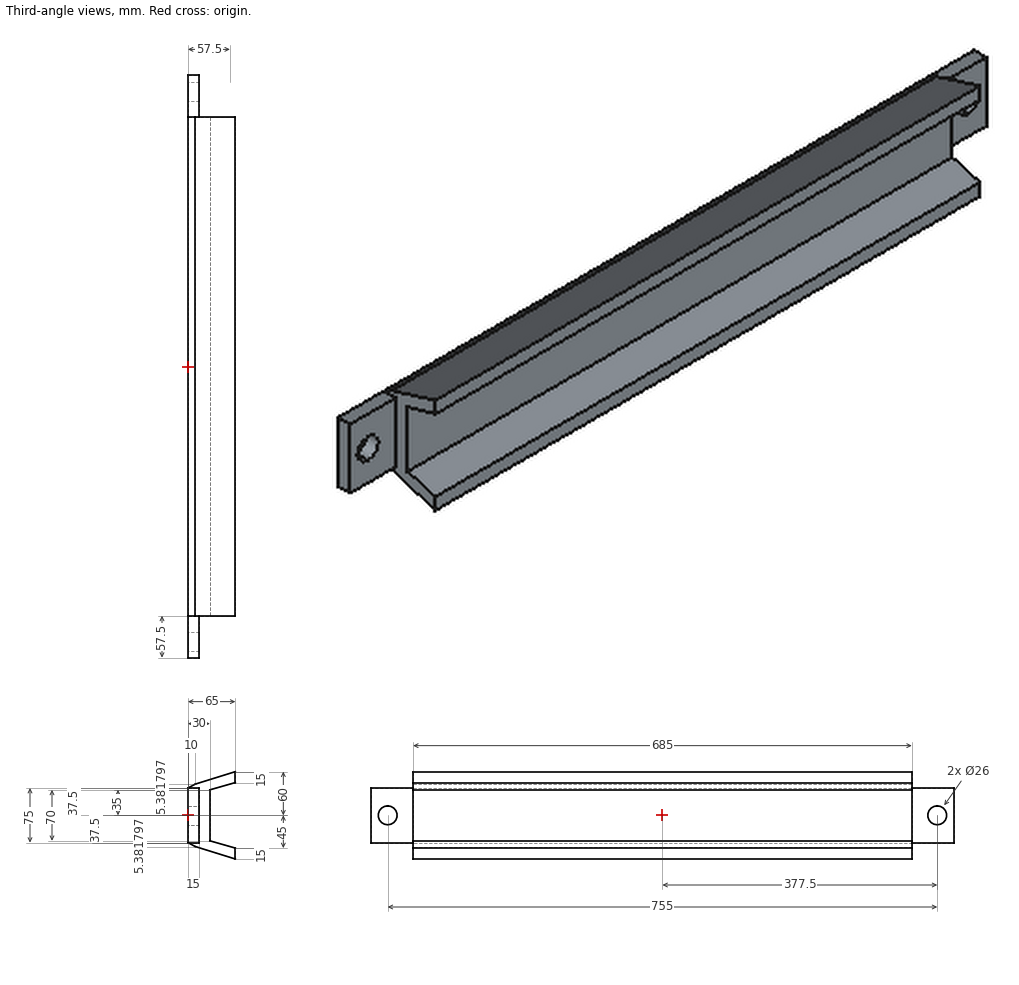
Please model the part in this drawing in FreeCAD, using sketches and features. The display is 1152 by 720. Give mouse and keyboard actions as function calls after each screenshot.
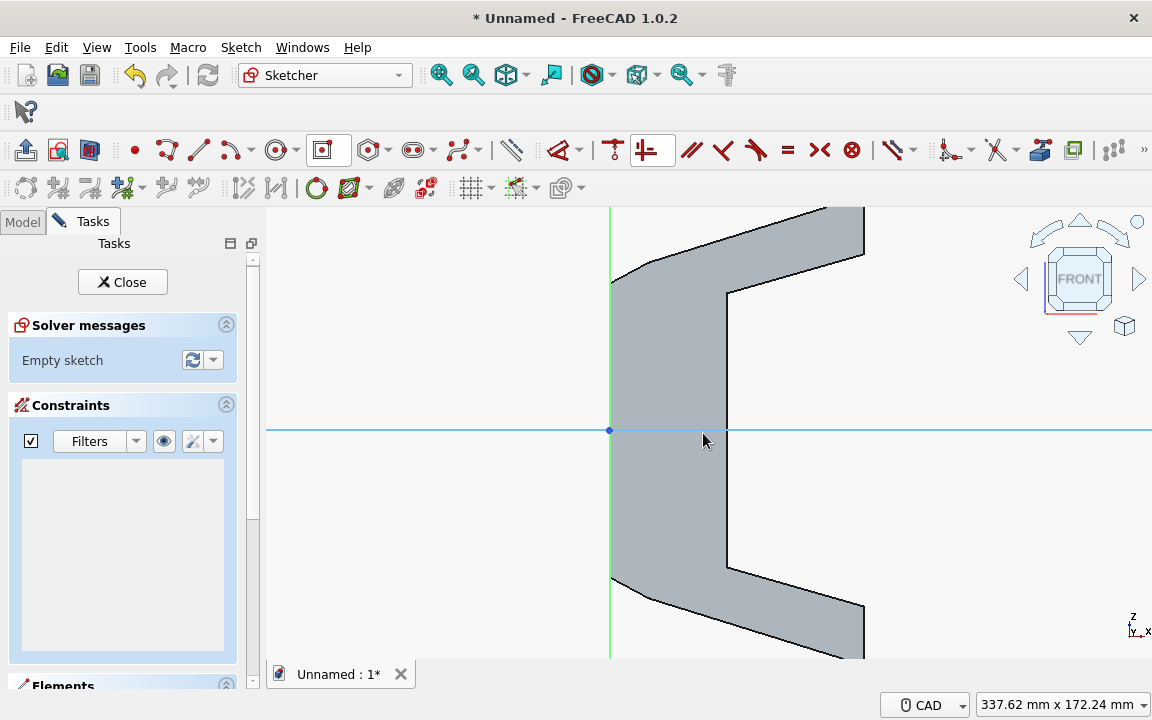
click(346, 150)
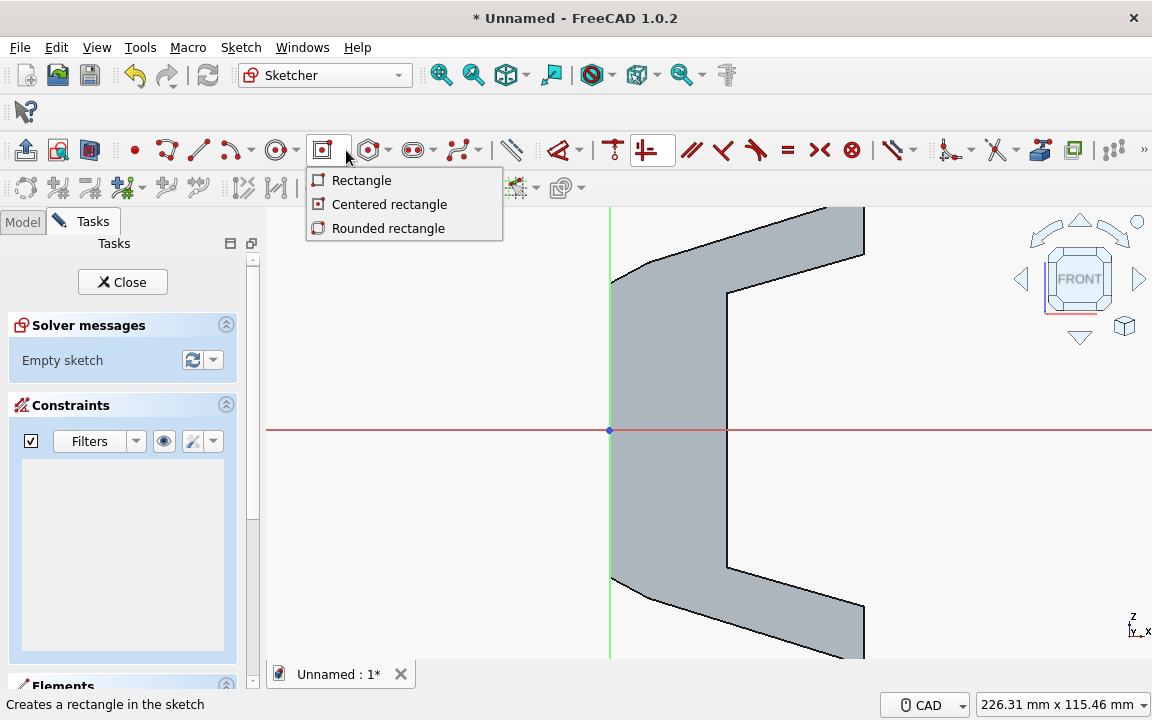
click(404, 180)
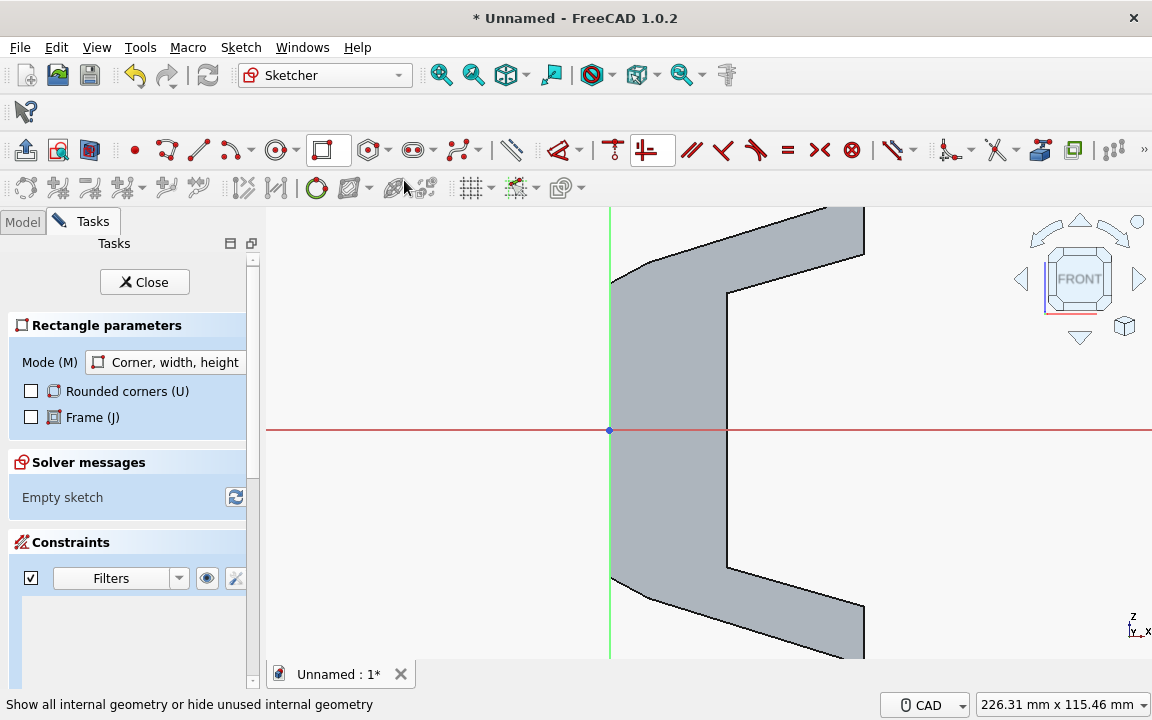
click(610, 284)
click(668, 577)
key(Escape)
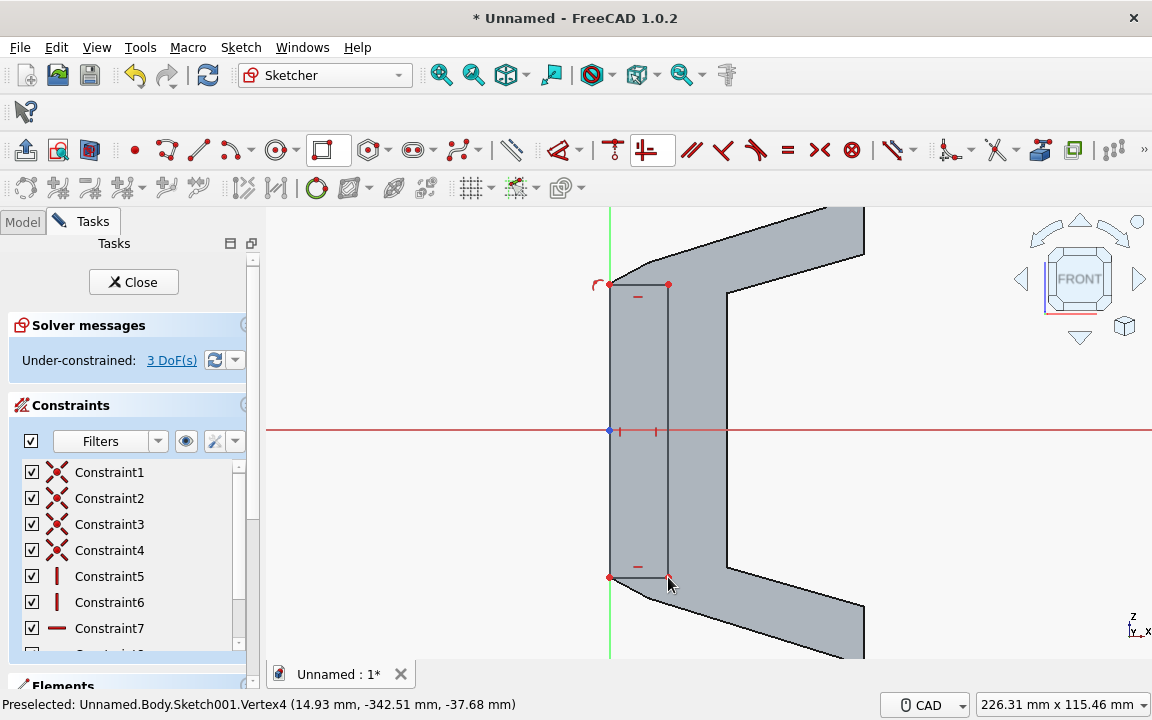
click(558, 150)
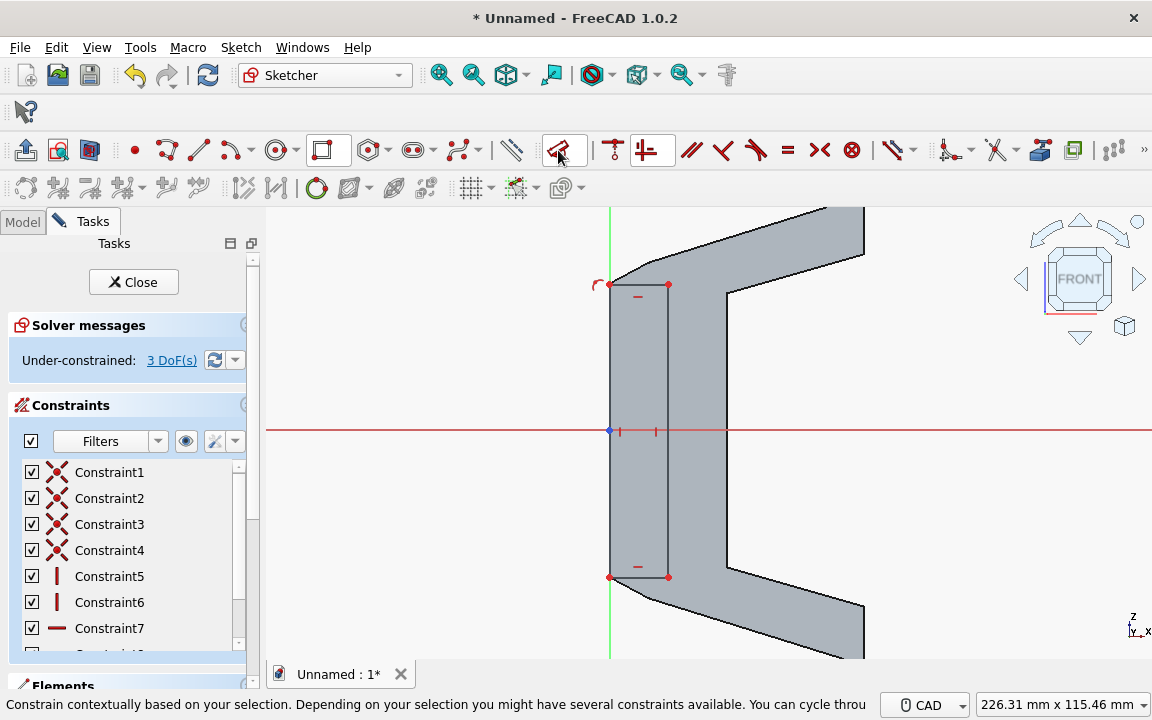
click(610, 373)
click(576, 364)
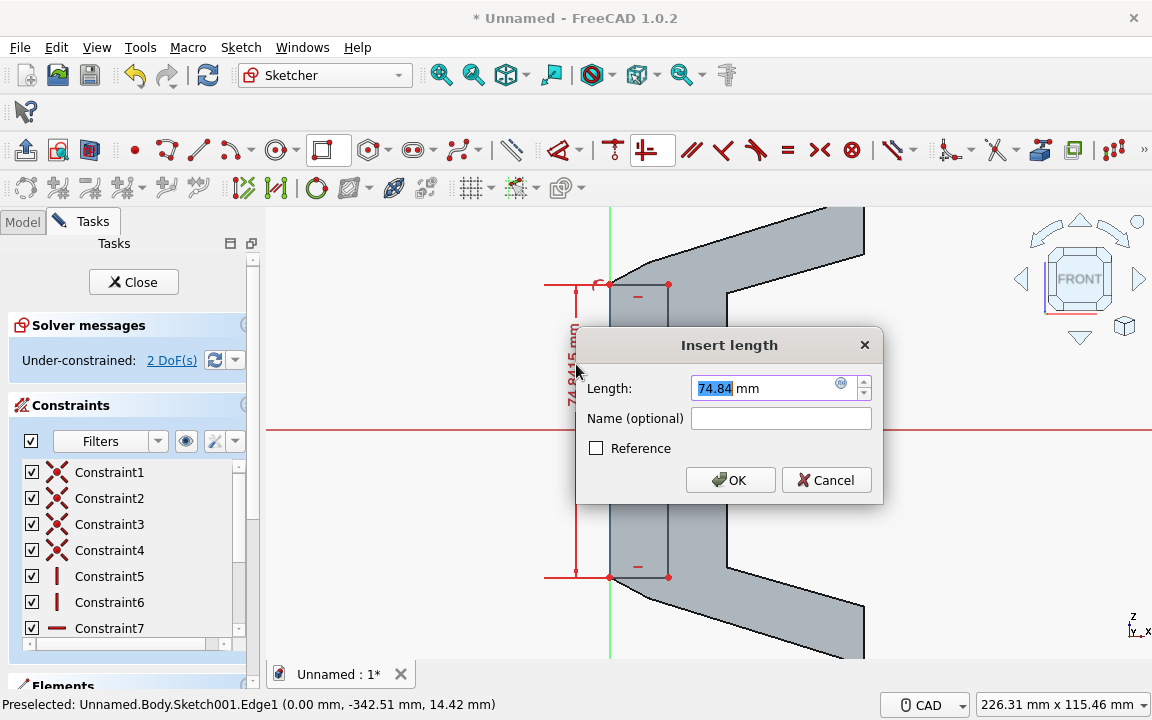
text(75)
key(Return)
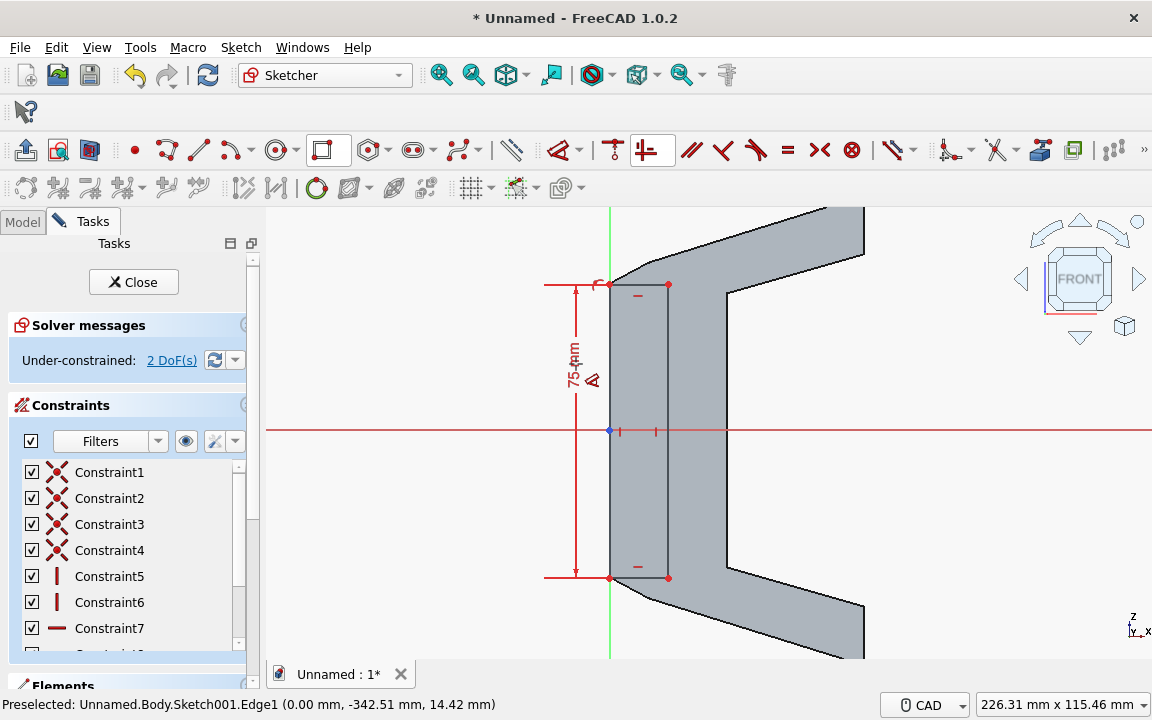
click(627, 578)
click(639, 612)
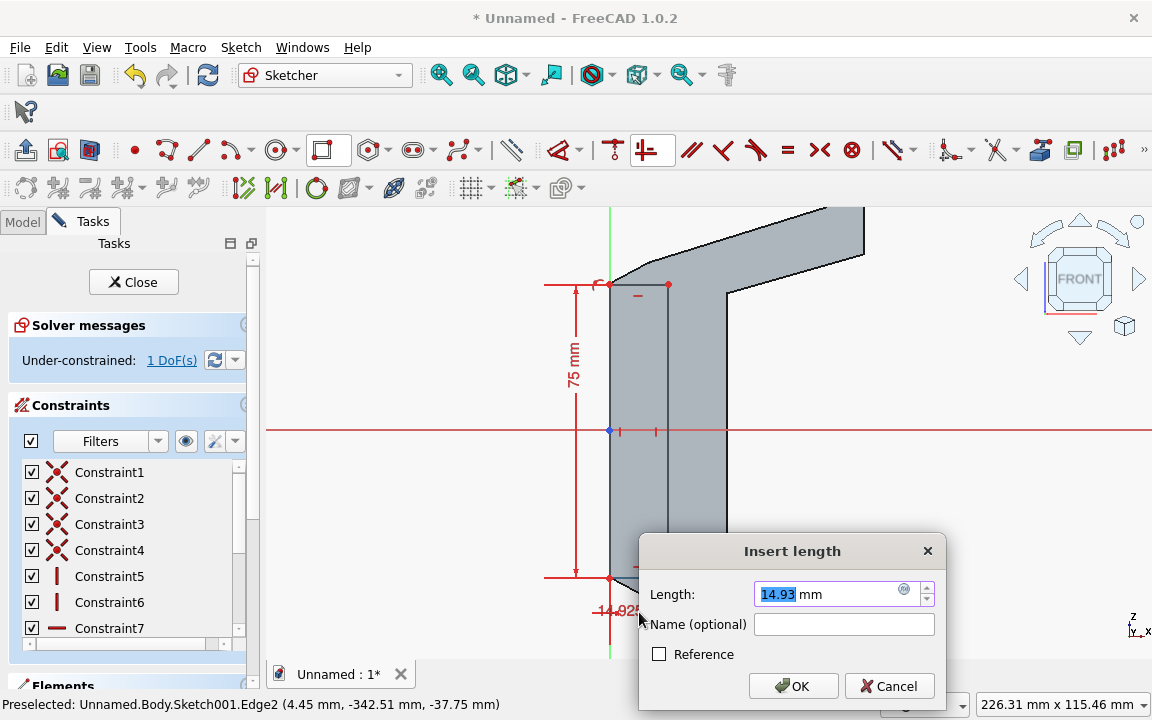
text(15)
key(Return)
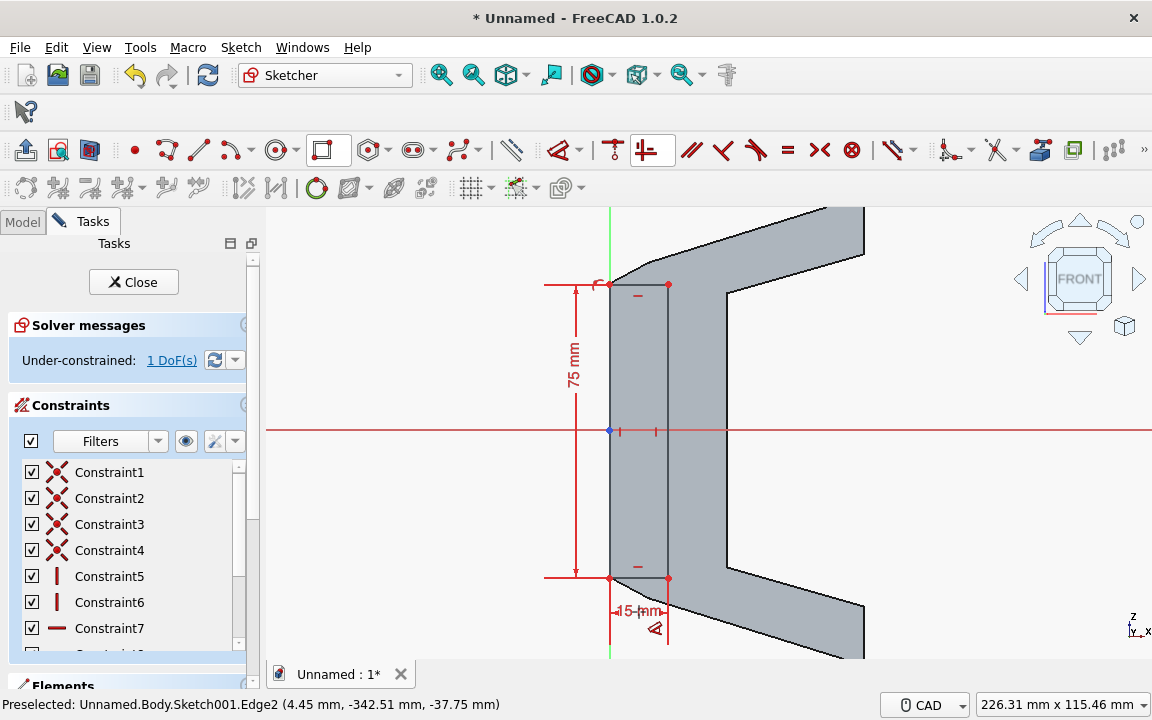
click(610, 285)
click(576, 324)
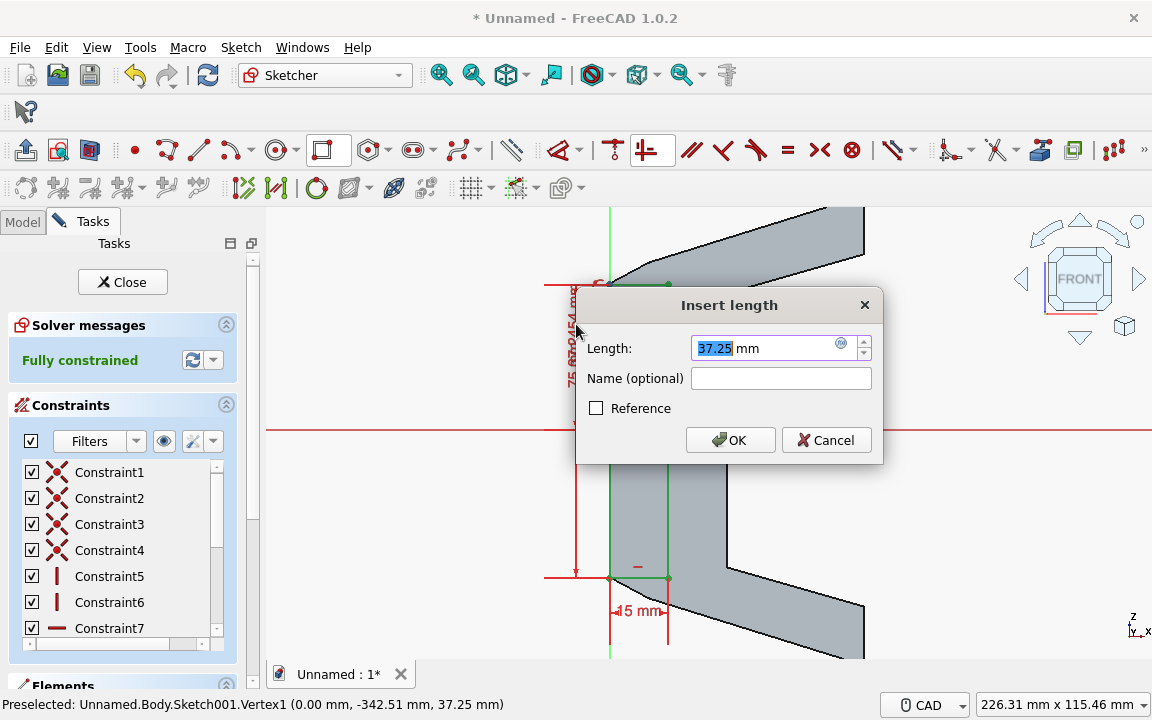
text(37.5)
key(Return)
key(Escape)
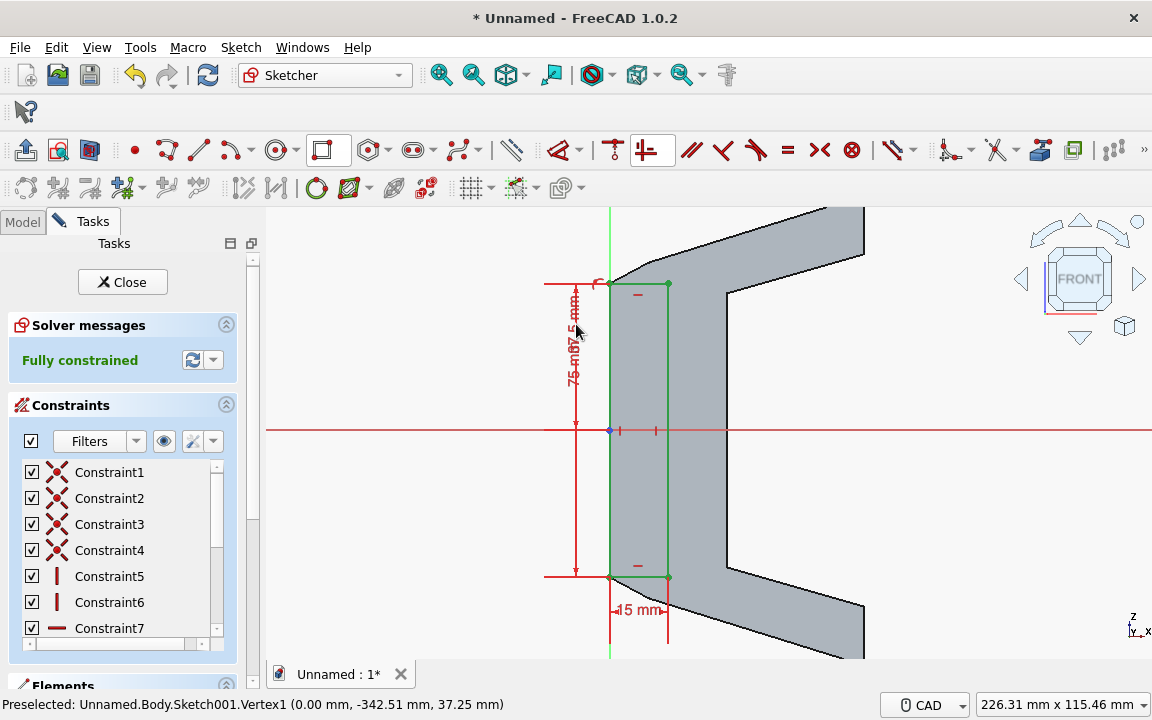
click(123, 282)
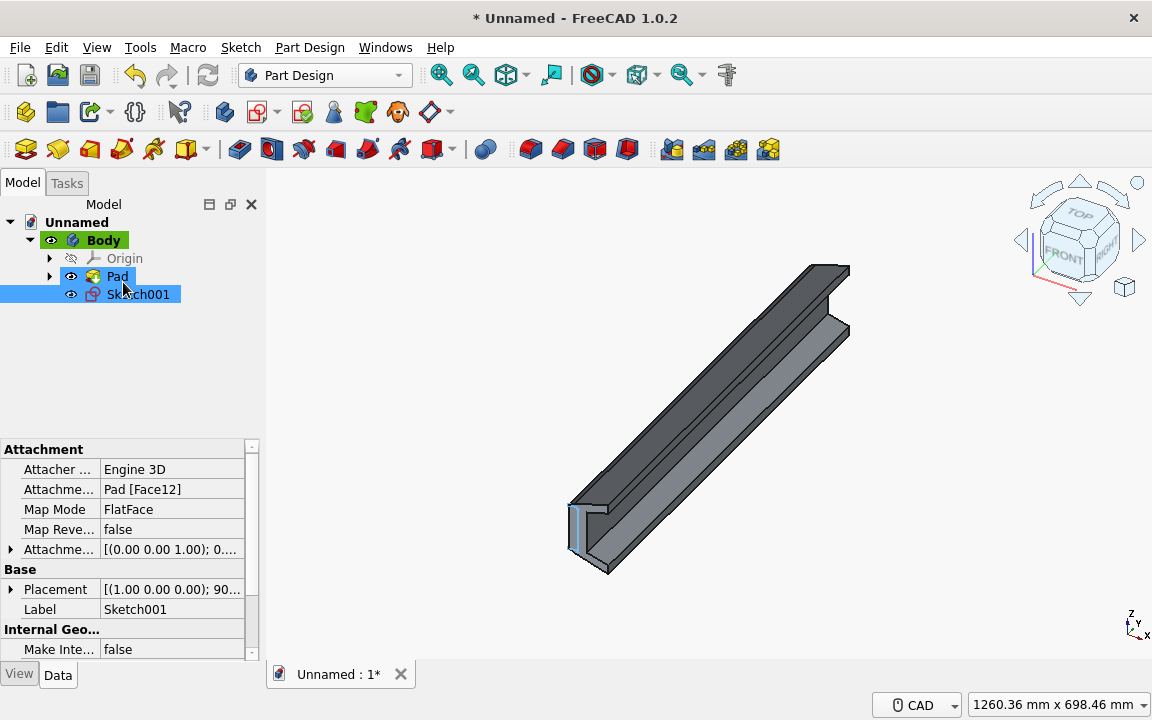
click(26, 150)